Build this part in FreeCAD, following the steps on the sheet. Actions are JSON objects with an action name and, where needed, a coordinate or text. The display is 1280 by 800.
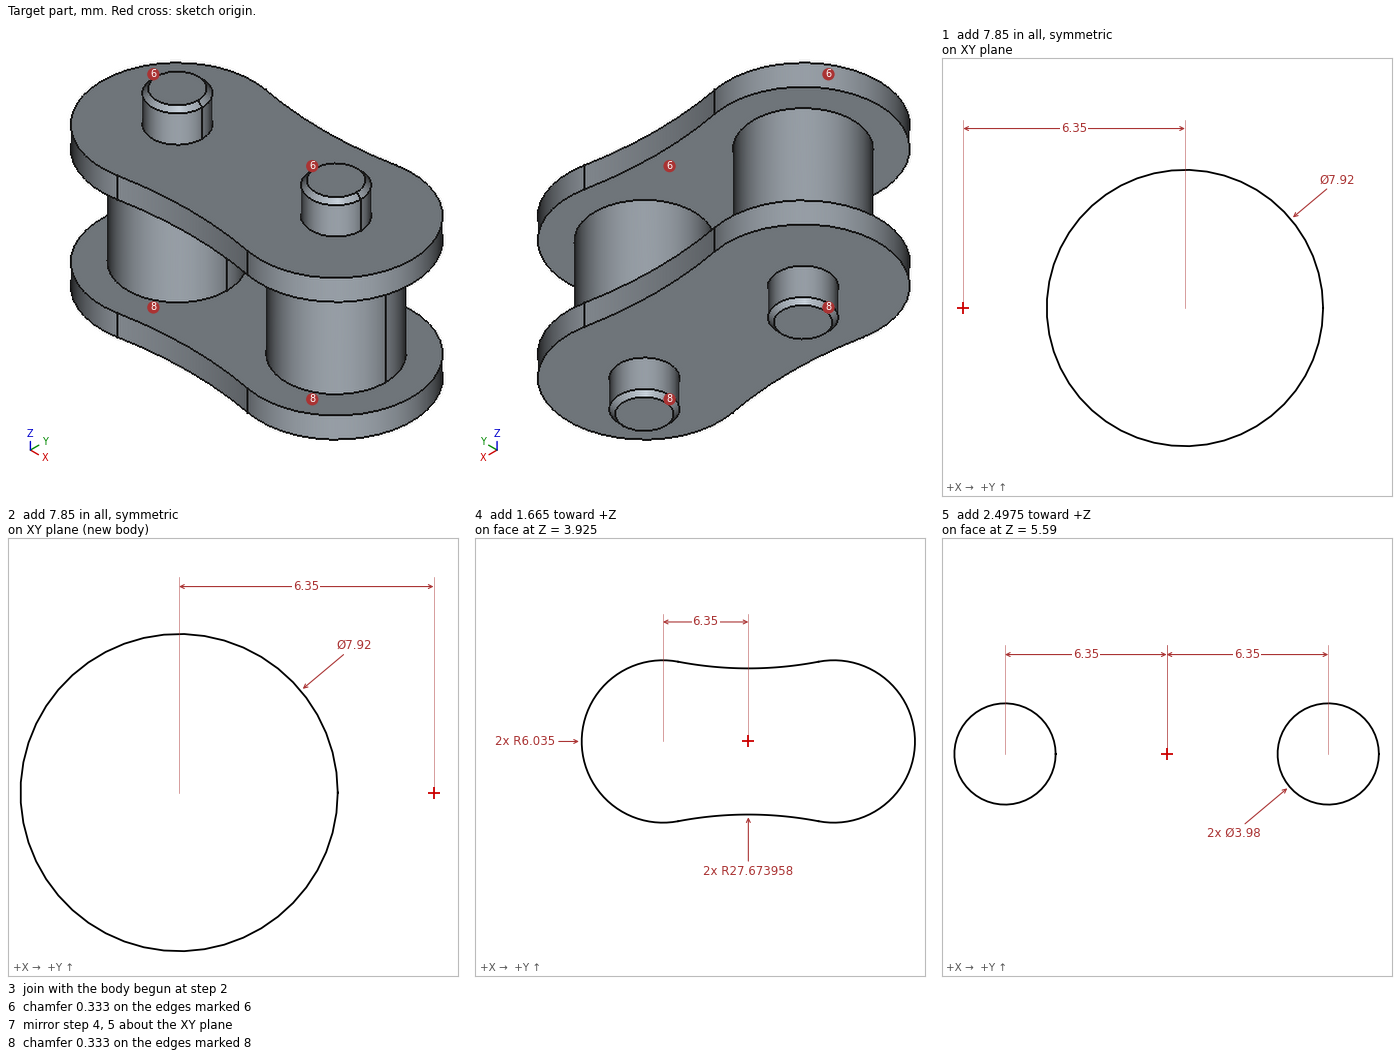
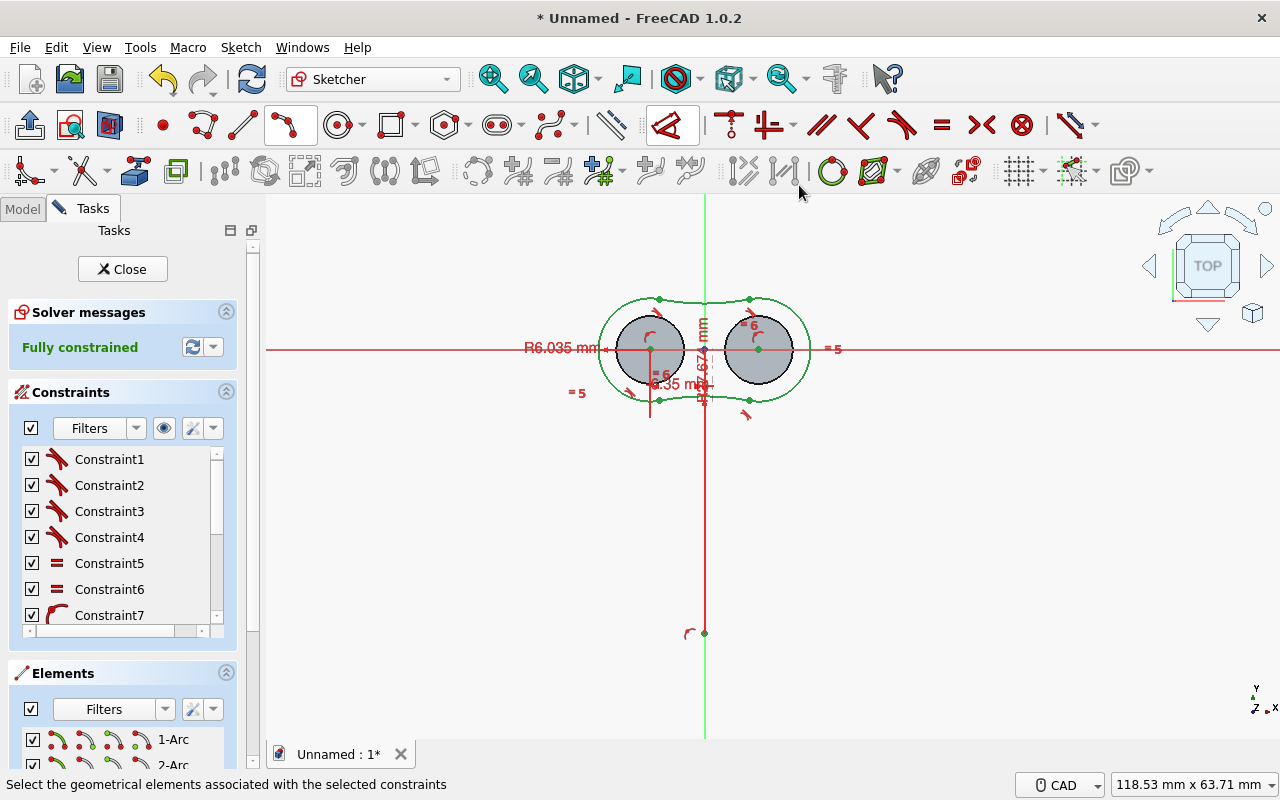
{"action": "left_click", "coordinate": [123, 269]}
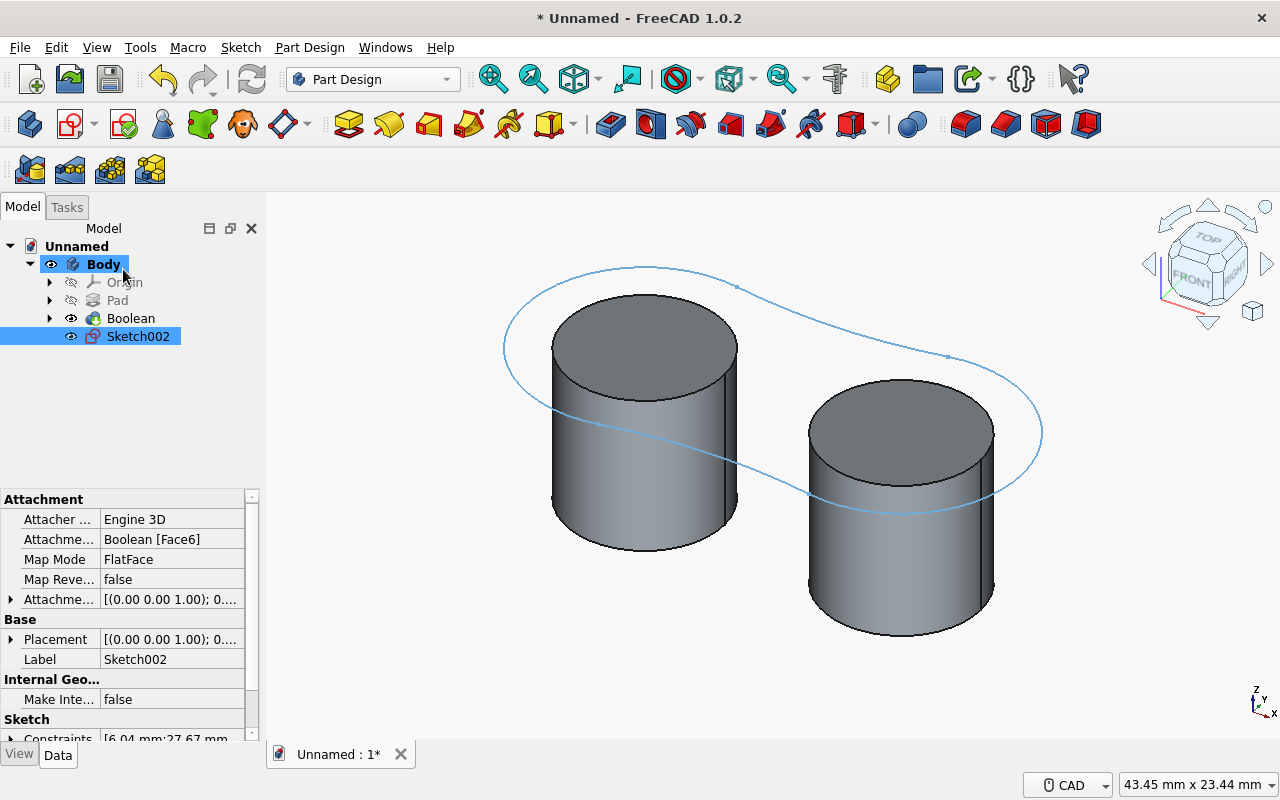
{"action": "left_click", "coordinate": [350, 124]}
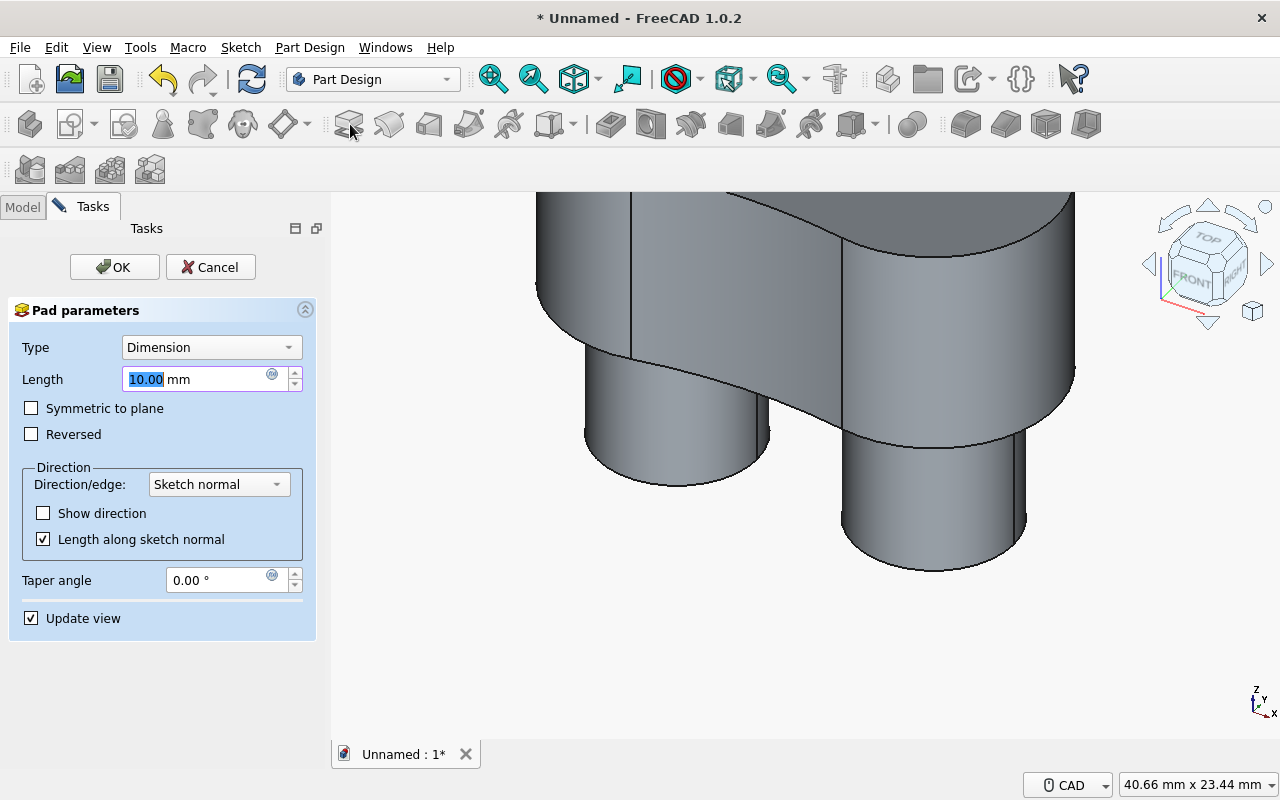
{"action": "type", "text": "1.665"}
{"action": "key", "text": "Tab"}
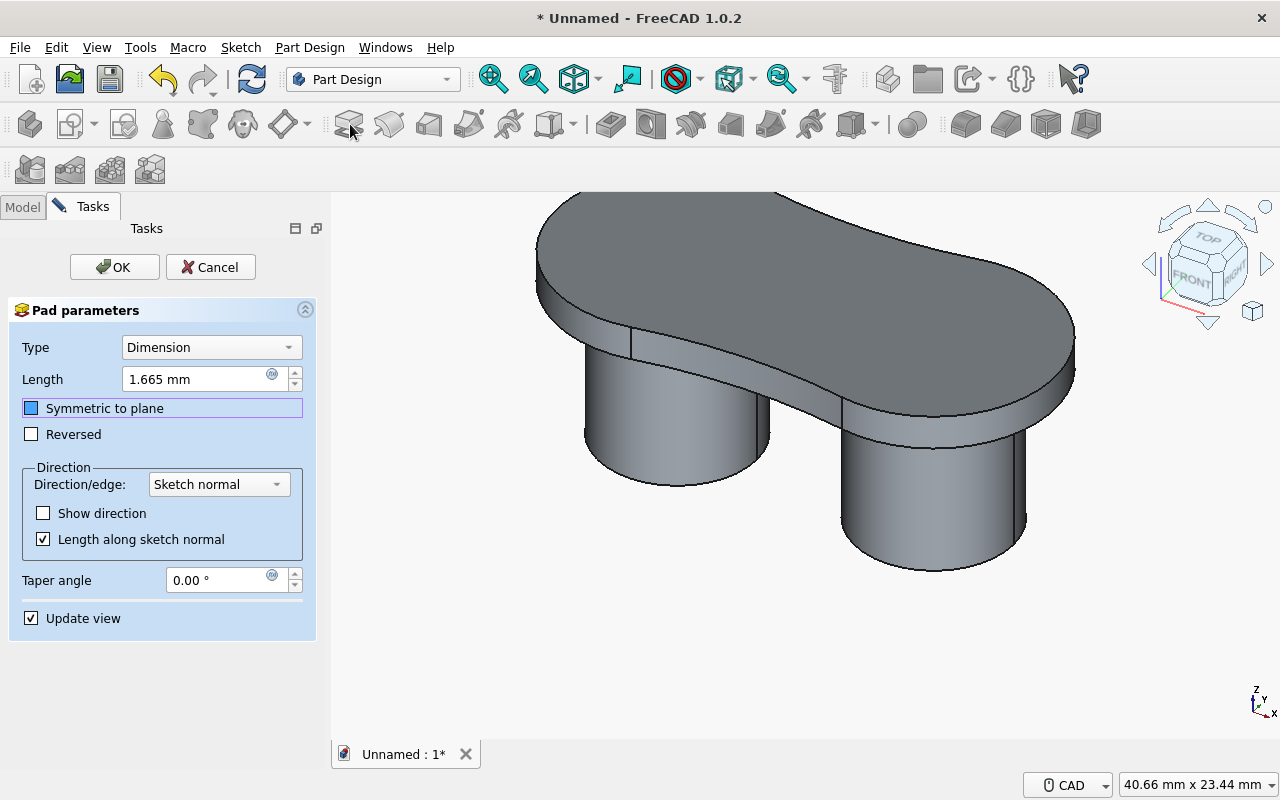
{"action": "left_click", "coordinate": [115, 267]}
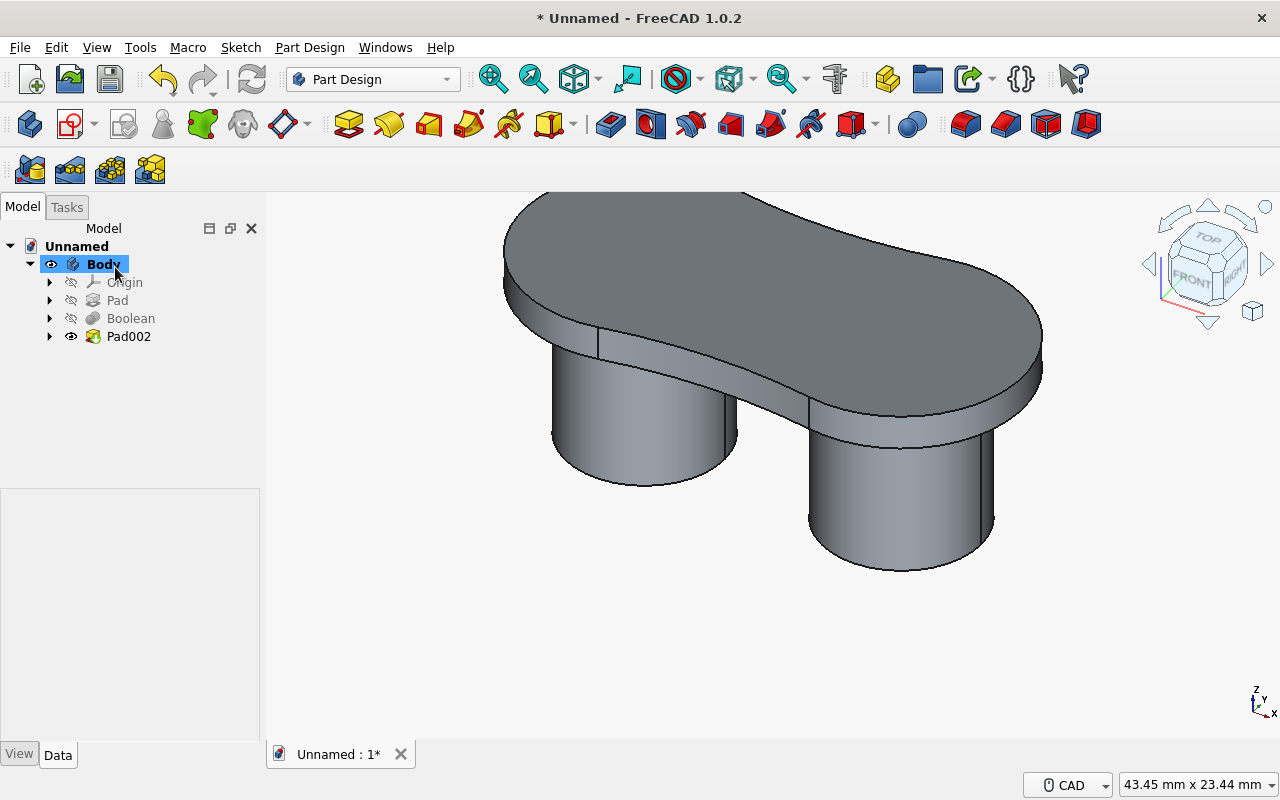
{"action": "left_click", "coordinate": [494, 80]}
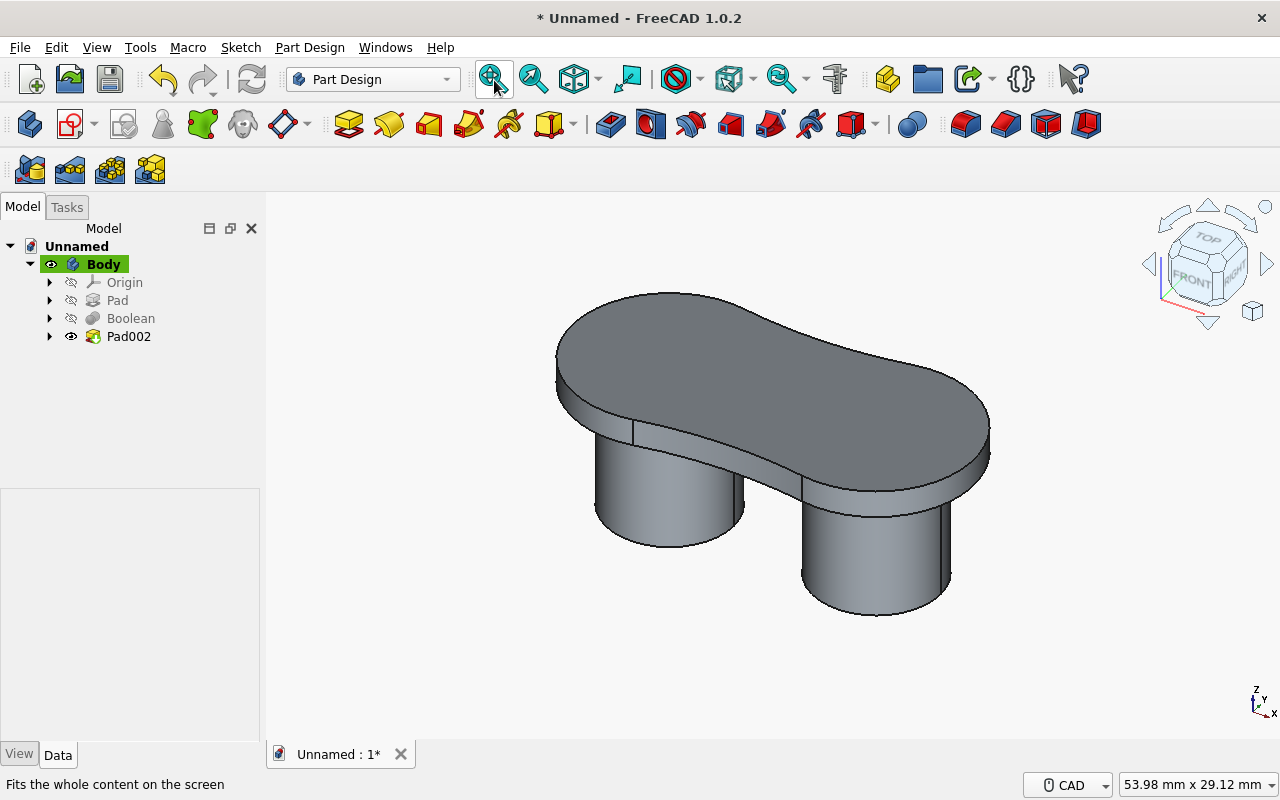
{"action": "left_click", "coordinate": [831, 410]}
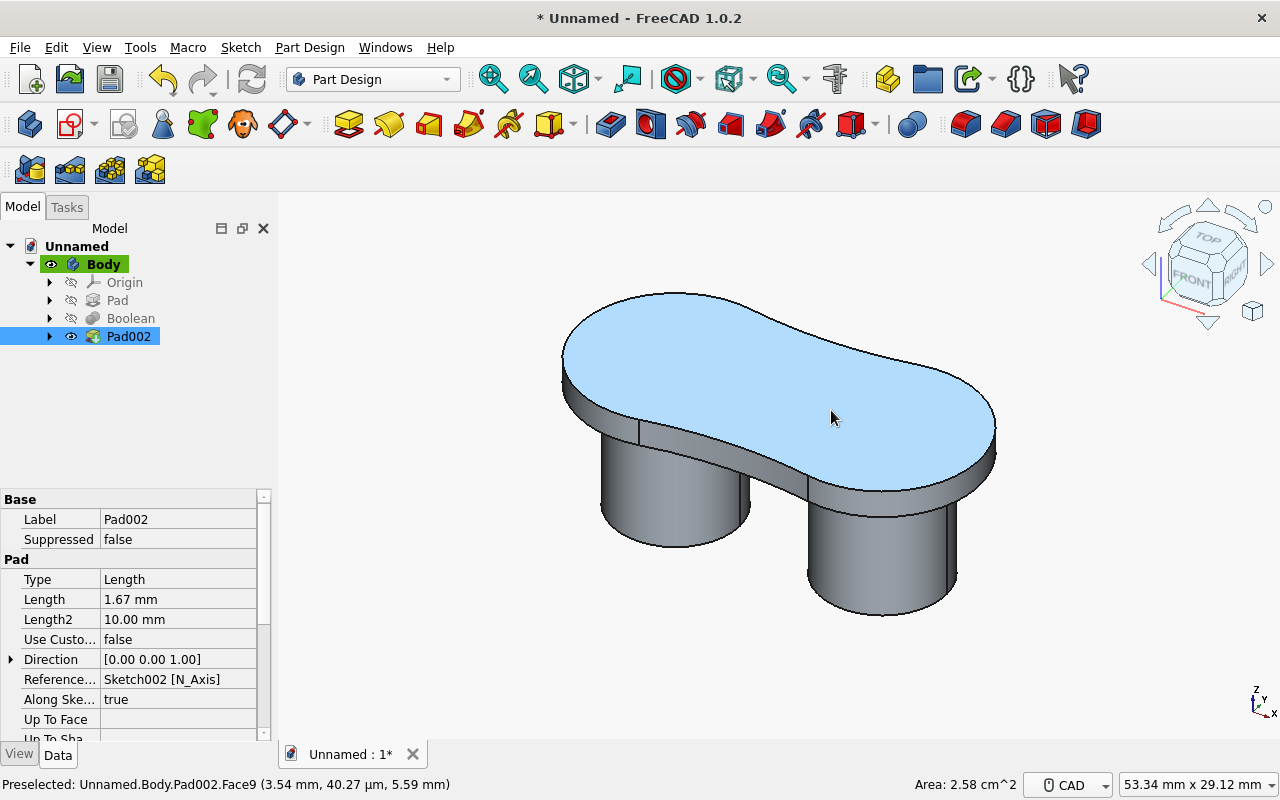
{"action": "left_click", "coordinate": [70, 124]}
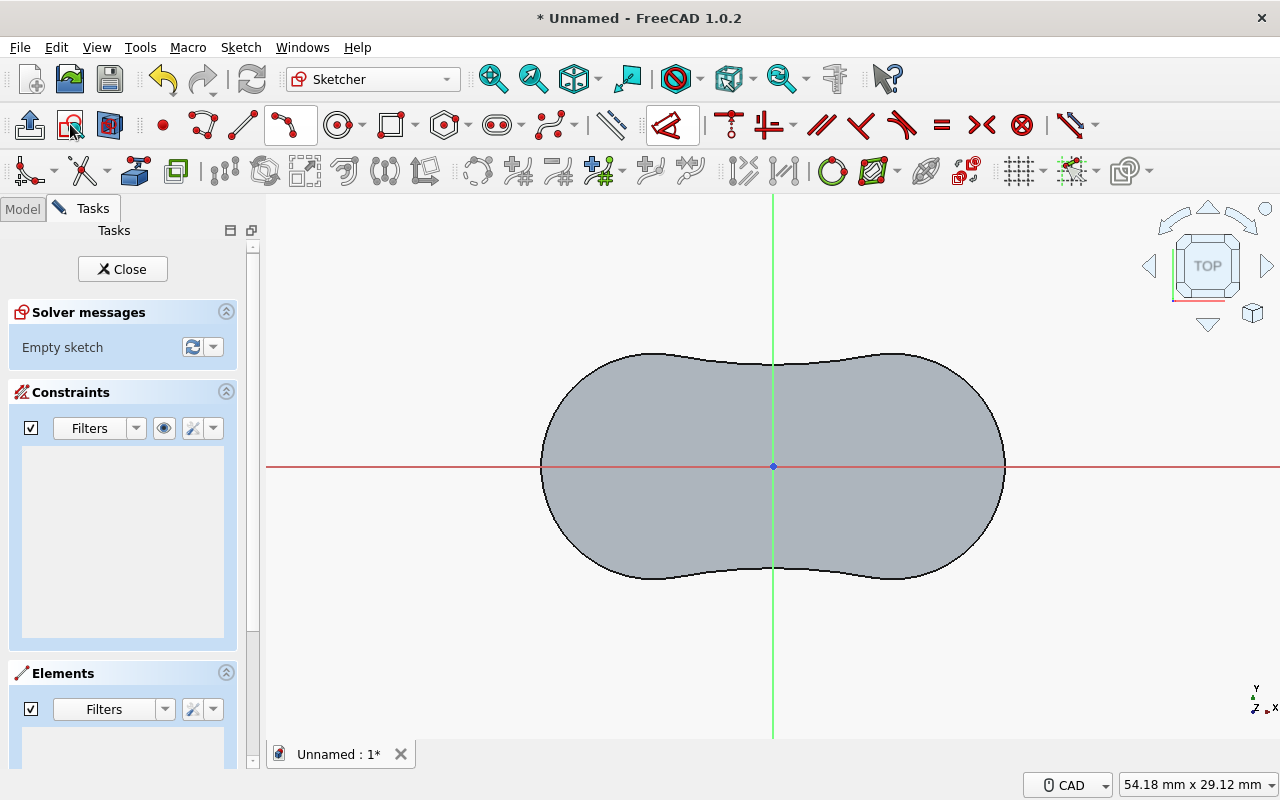
{"action": "scroll", "coordinate": [856, 466], "scroll_direction": "up", "scroll_amount": 3}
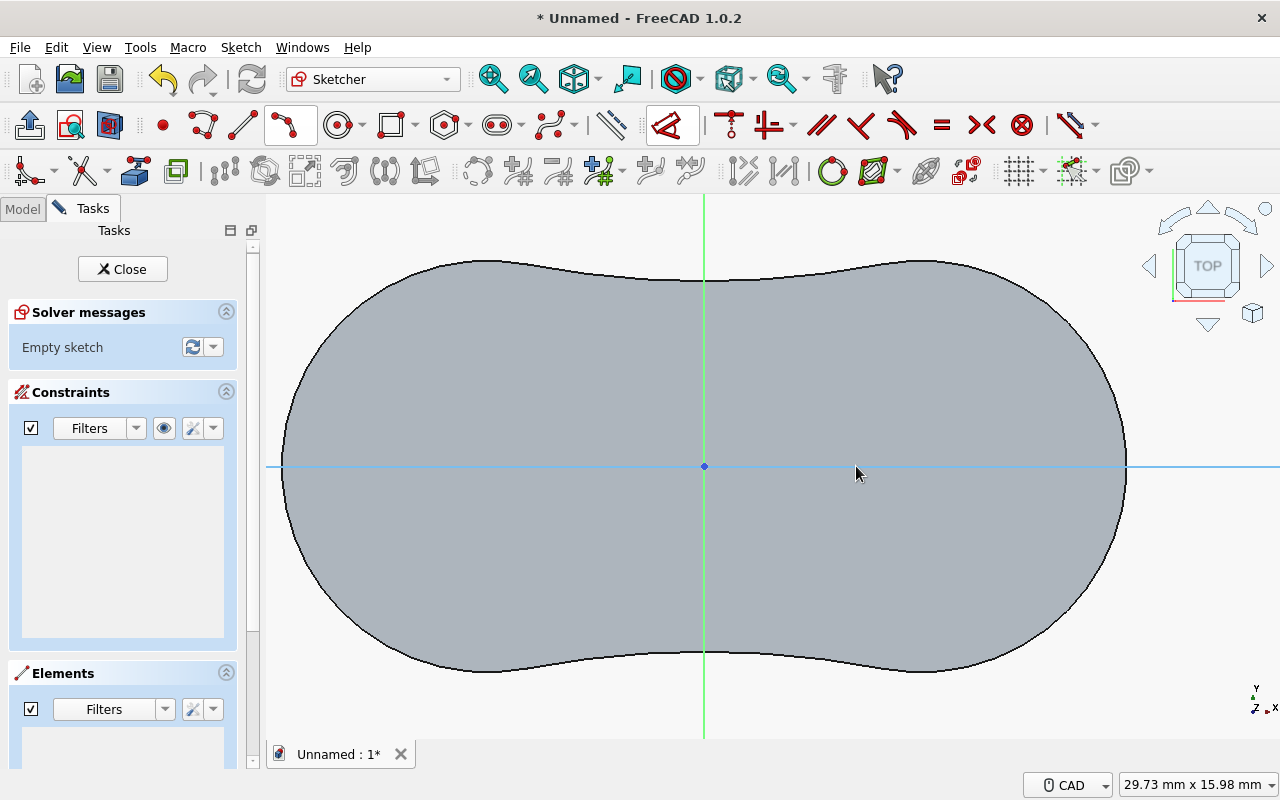
{"action": "left_click", "coordinate": [338, 126]}